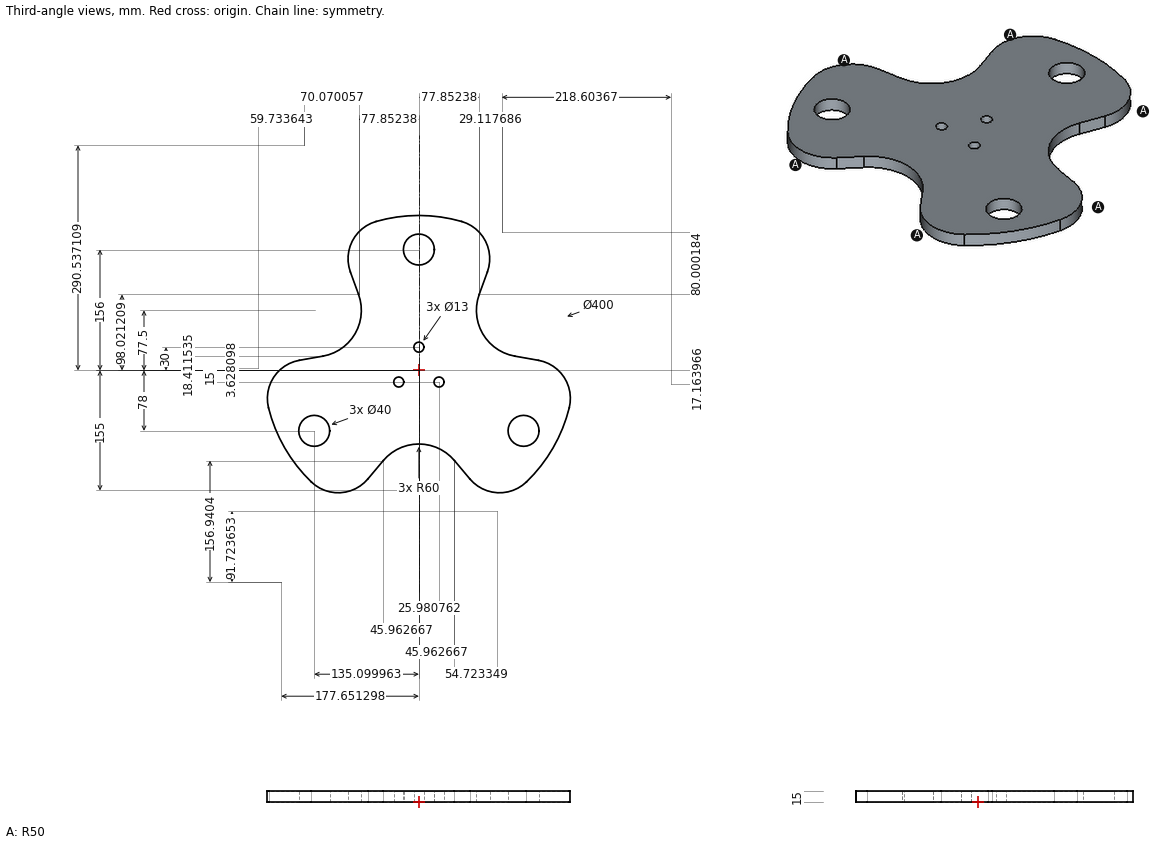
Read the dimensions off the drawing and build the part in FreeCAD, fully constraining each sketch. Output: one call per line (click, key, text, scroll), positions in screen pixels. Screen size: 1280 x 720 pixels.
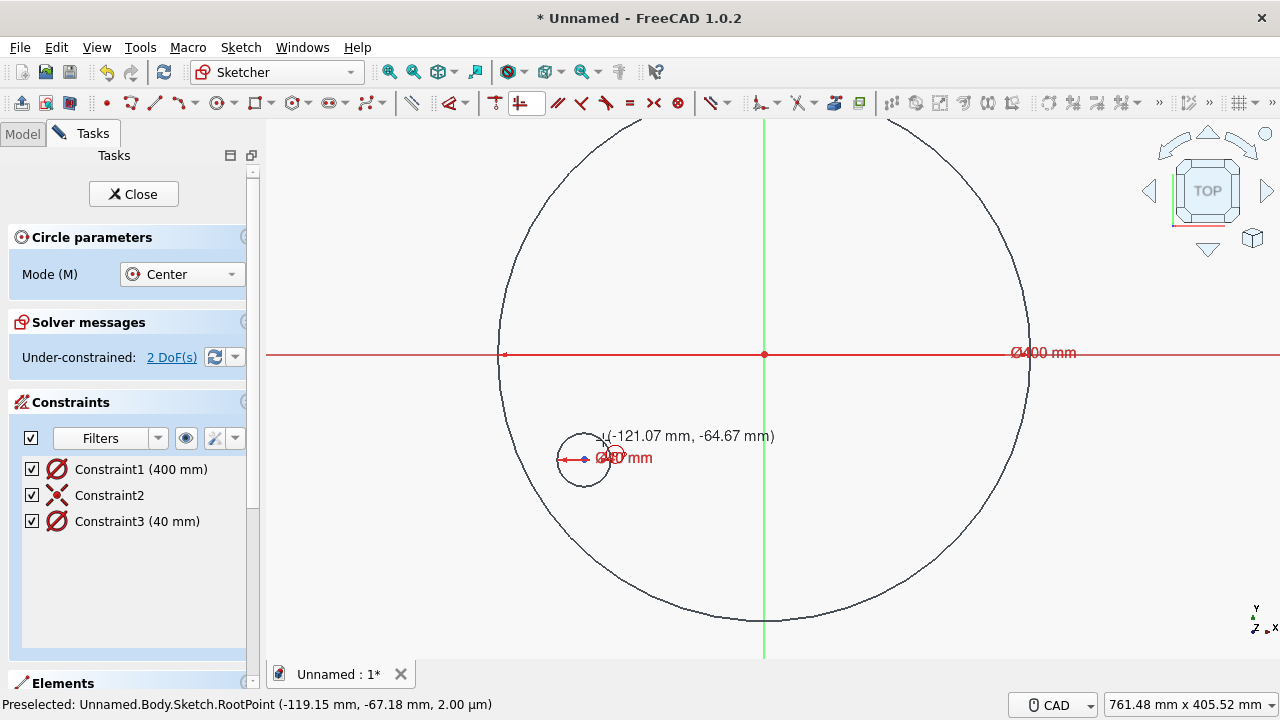
click(944, 459)
move(963, 440)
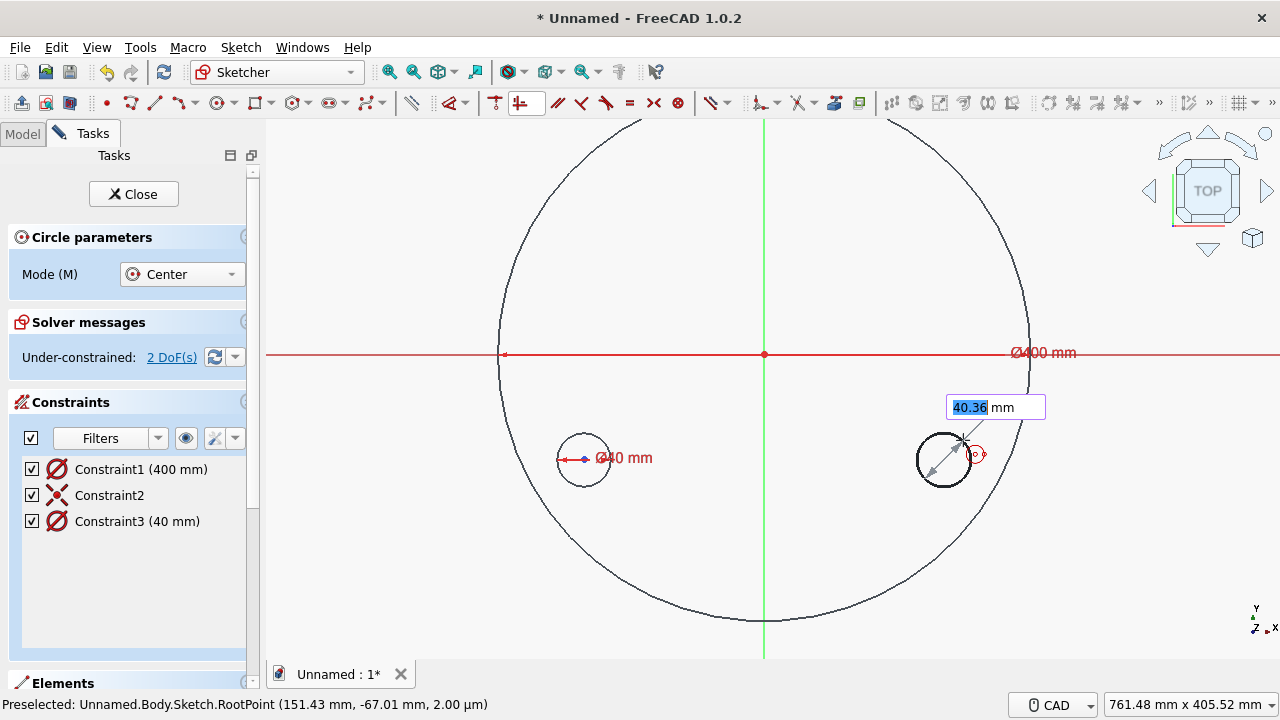
text(40)
key(Return)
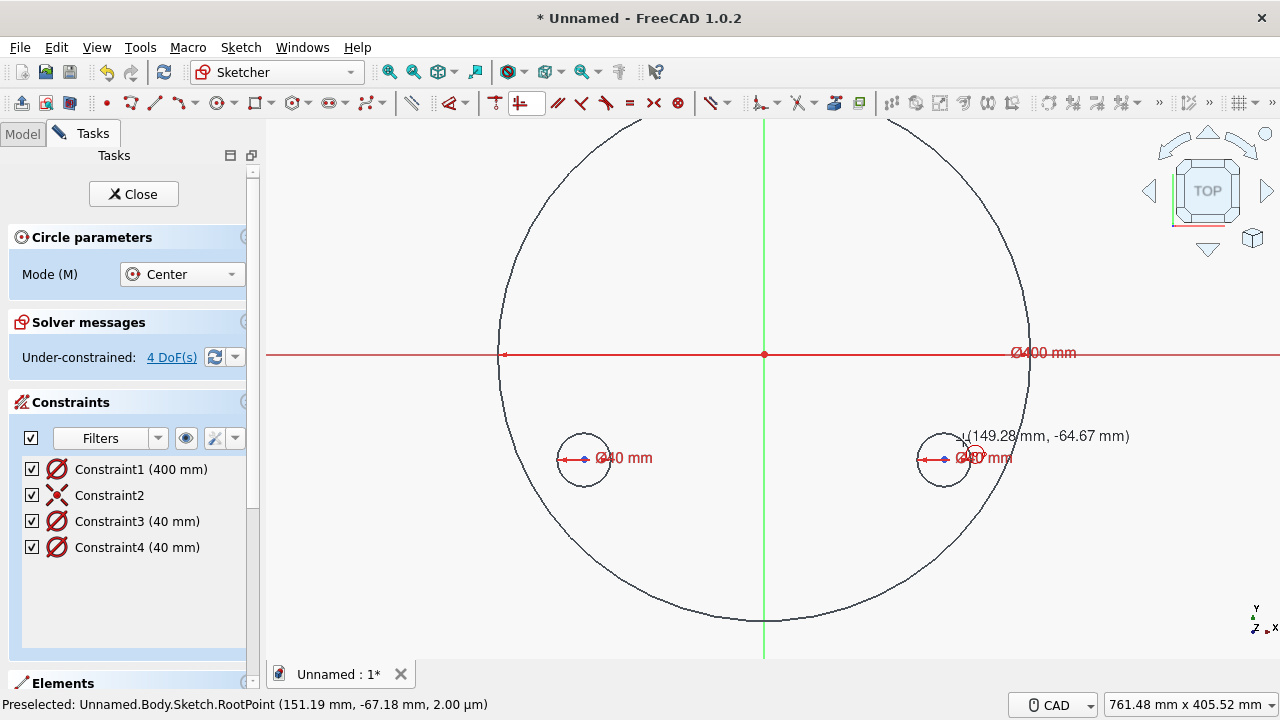
click(764, 147)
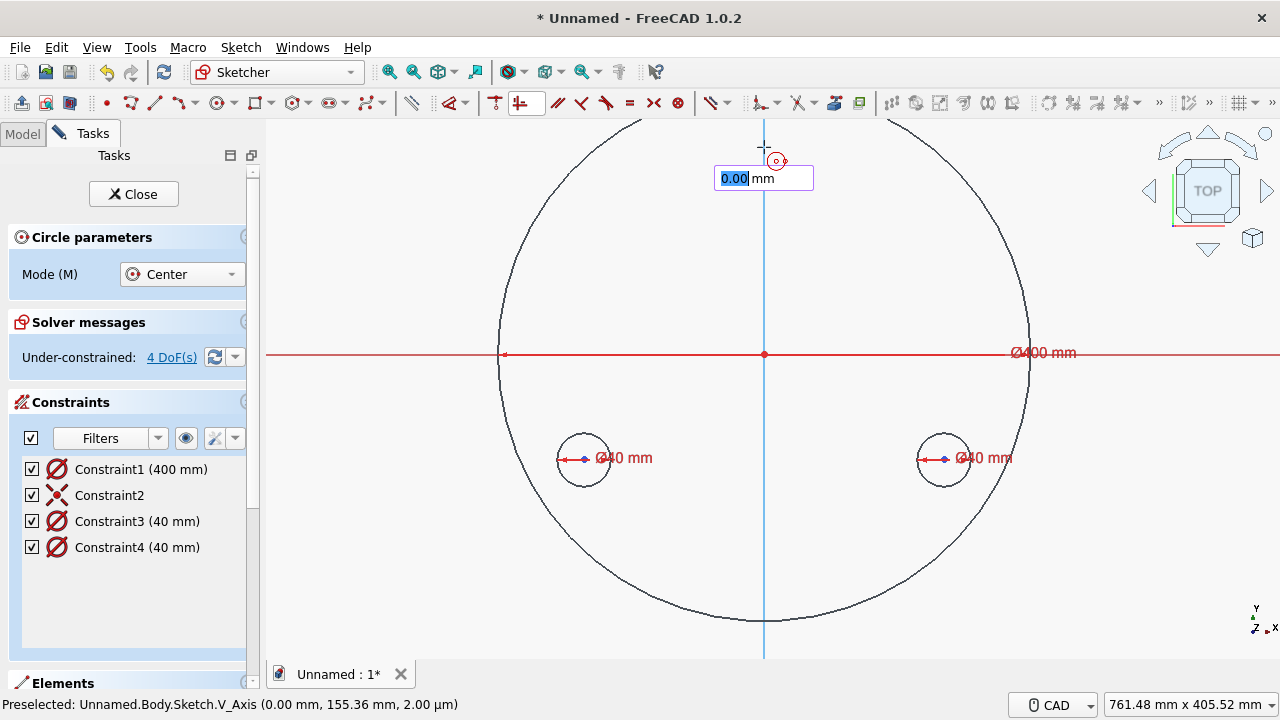
scroll(583, 458, down, 2)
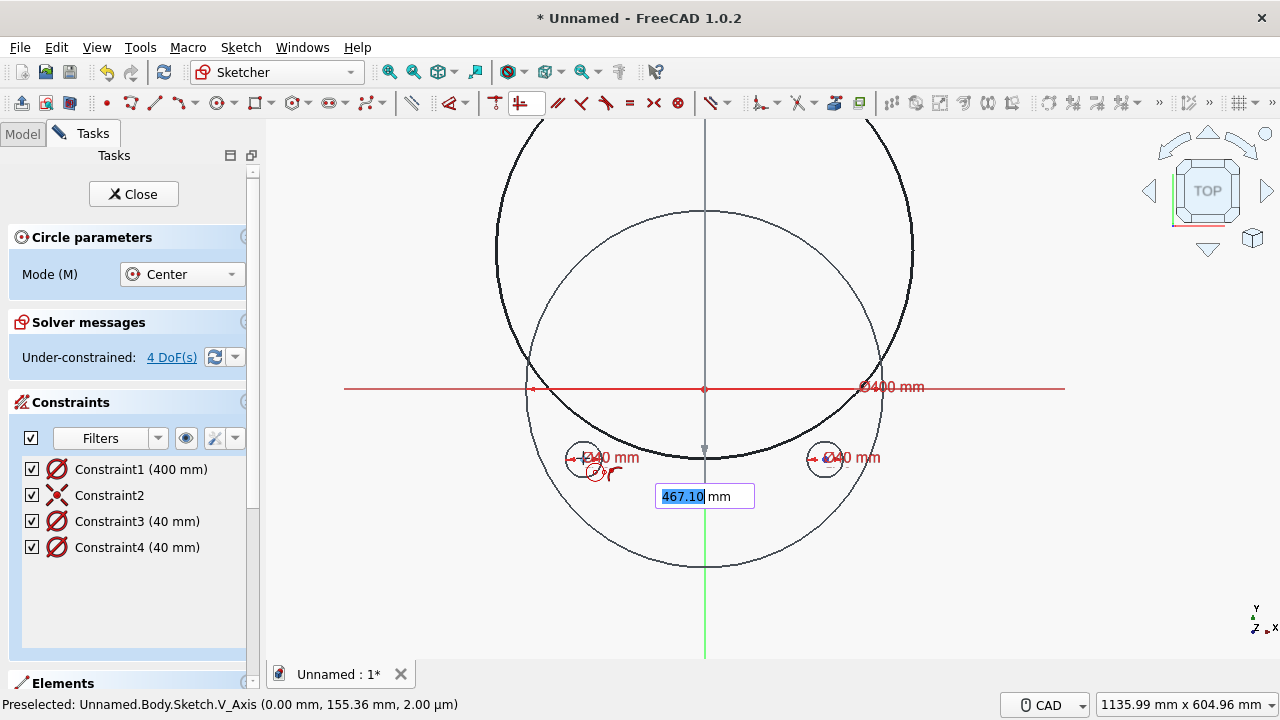
scroll(717, 237, up, 2)
move(717, 237)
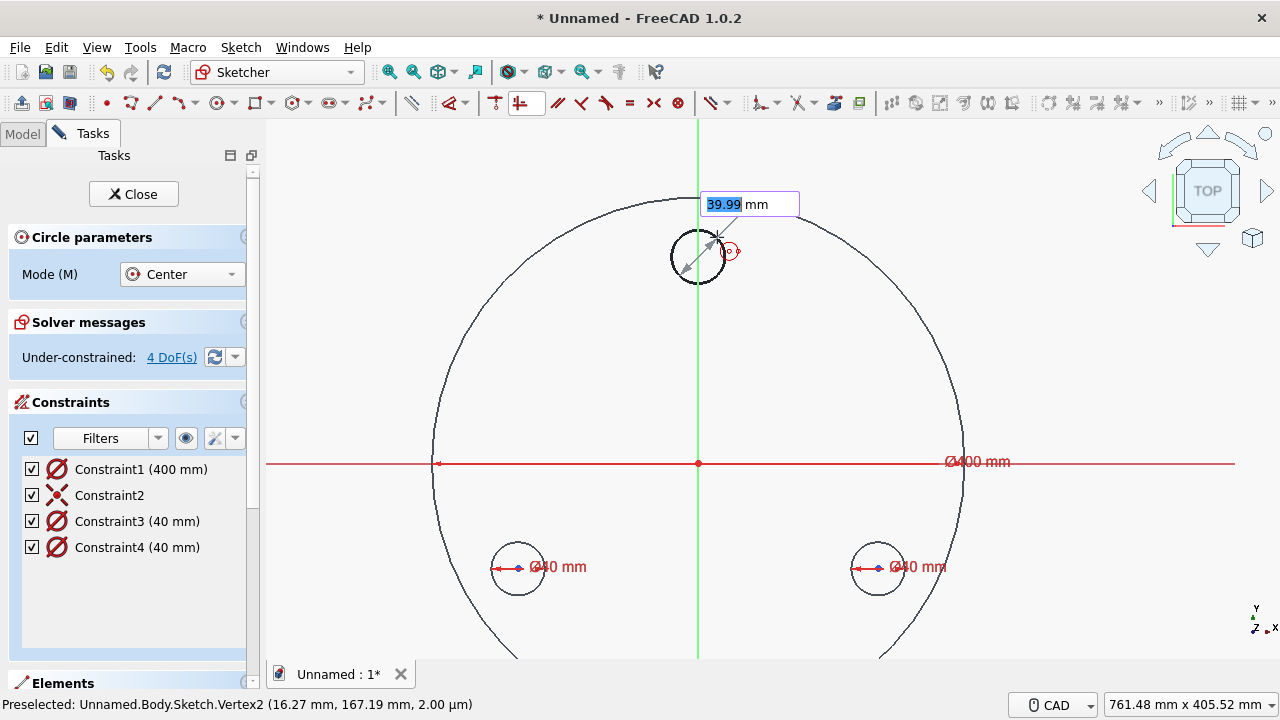
text(40)
key(Return)
key(Escape)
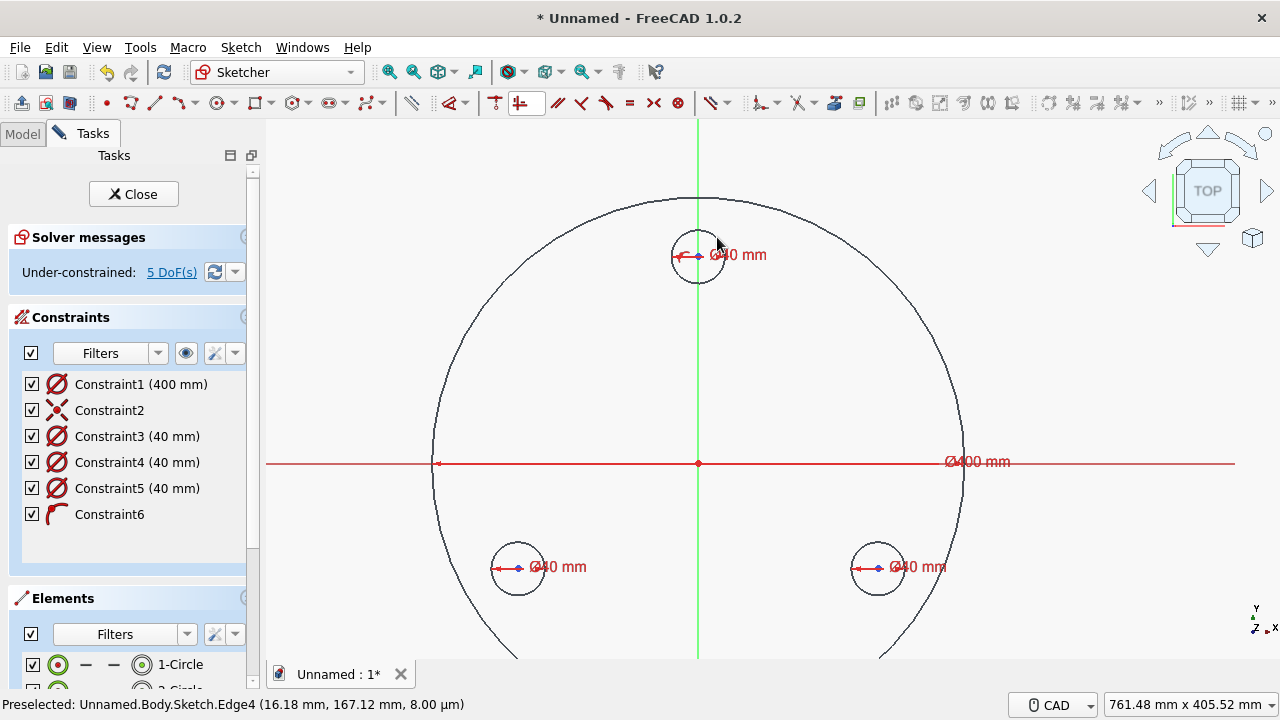
click(518, 569)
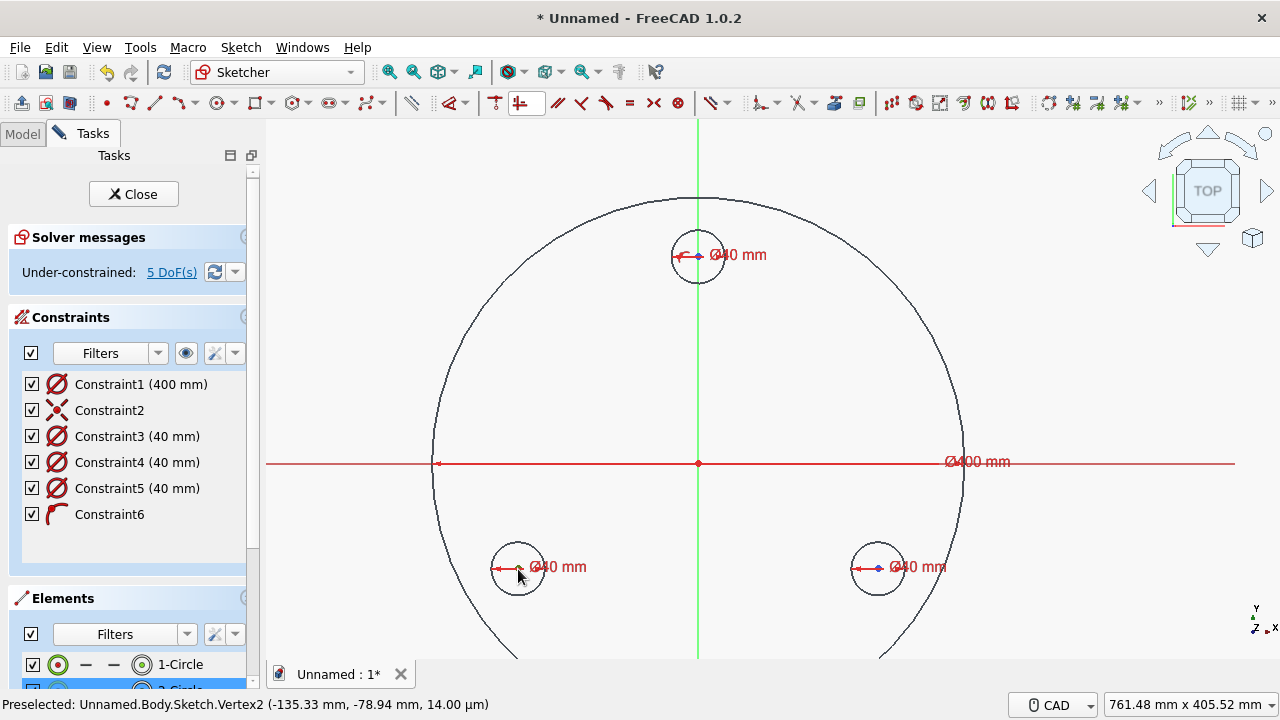
click(878, 569)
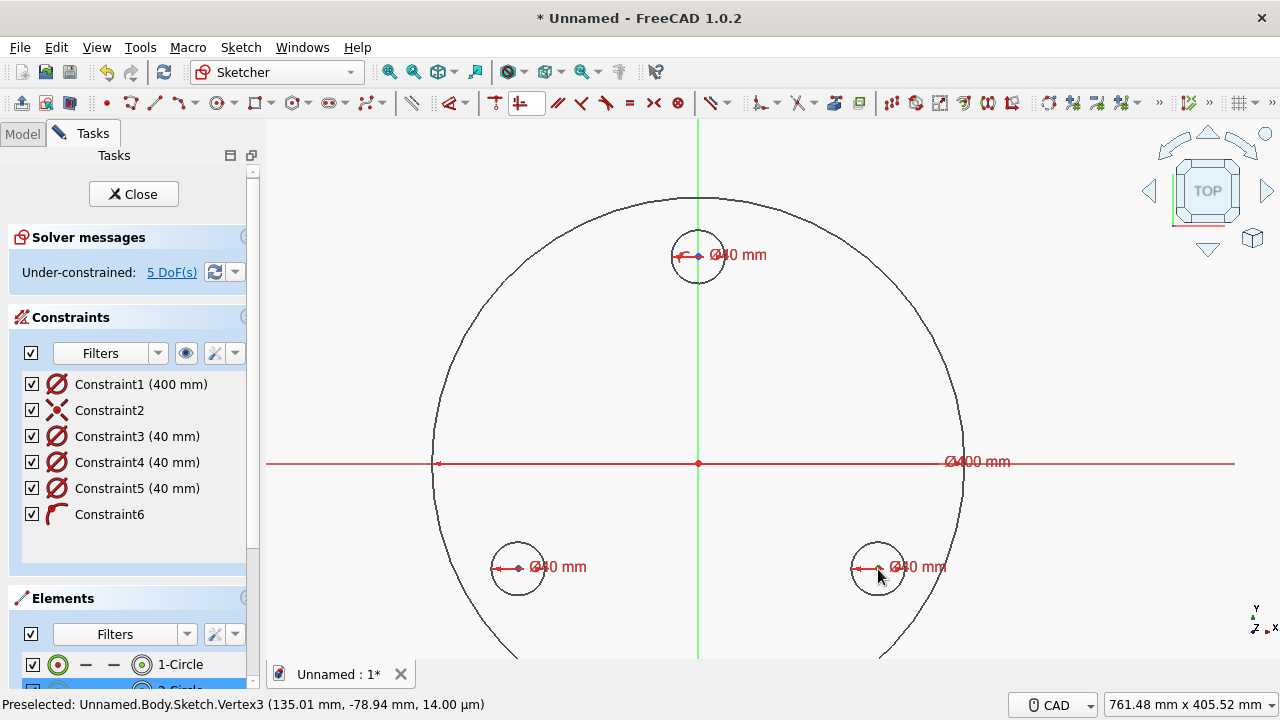
click(698, 596)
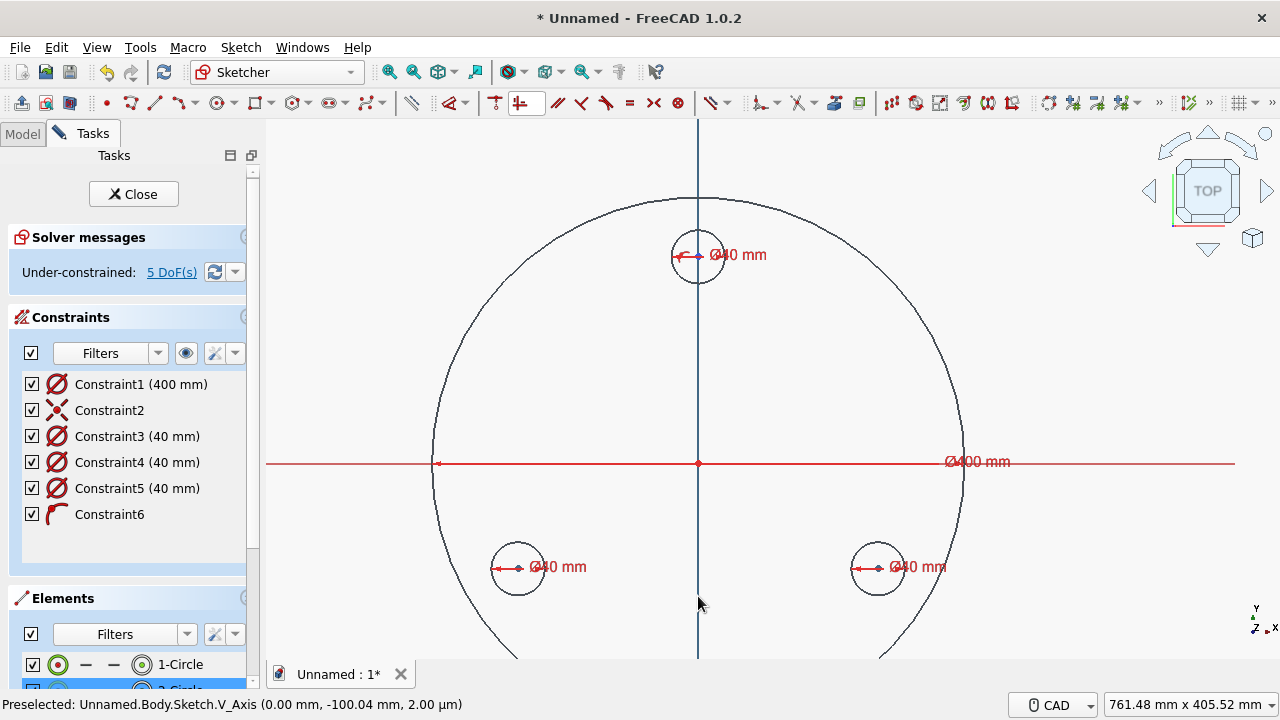
click(654, 104)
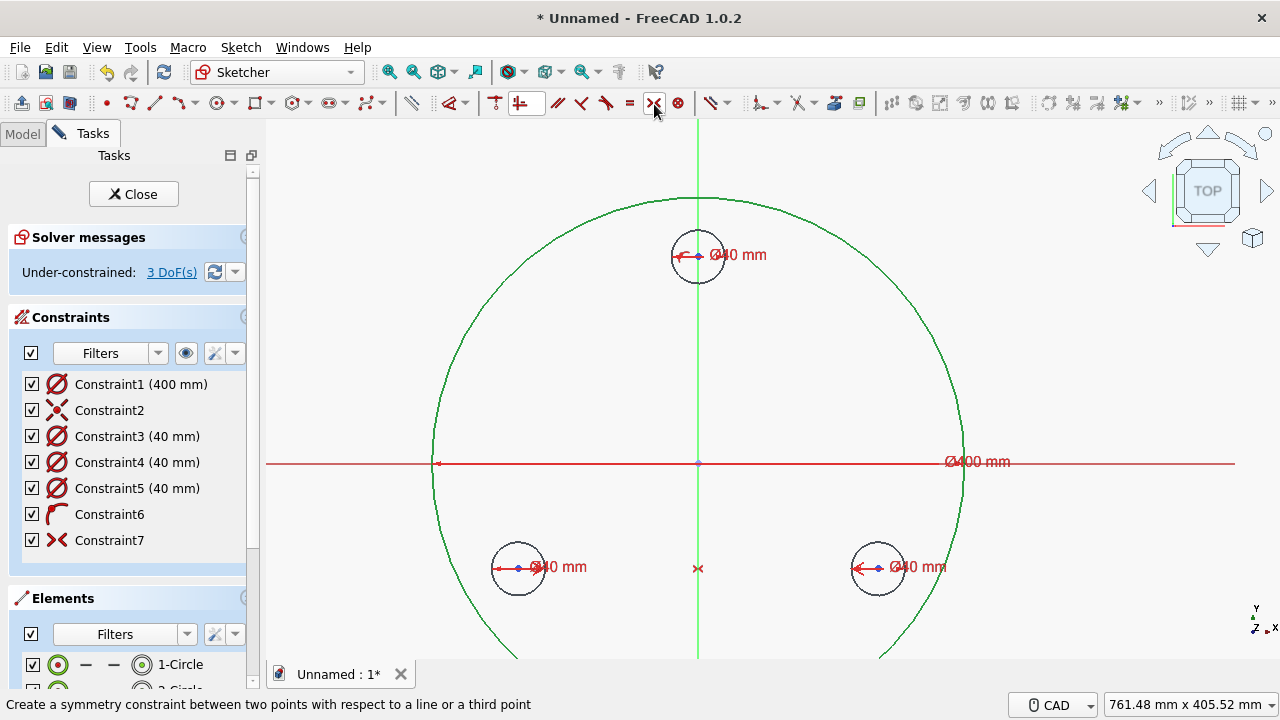
click(518, 569)